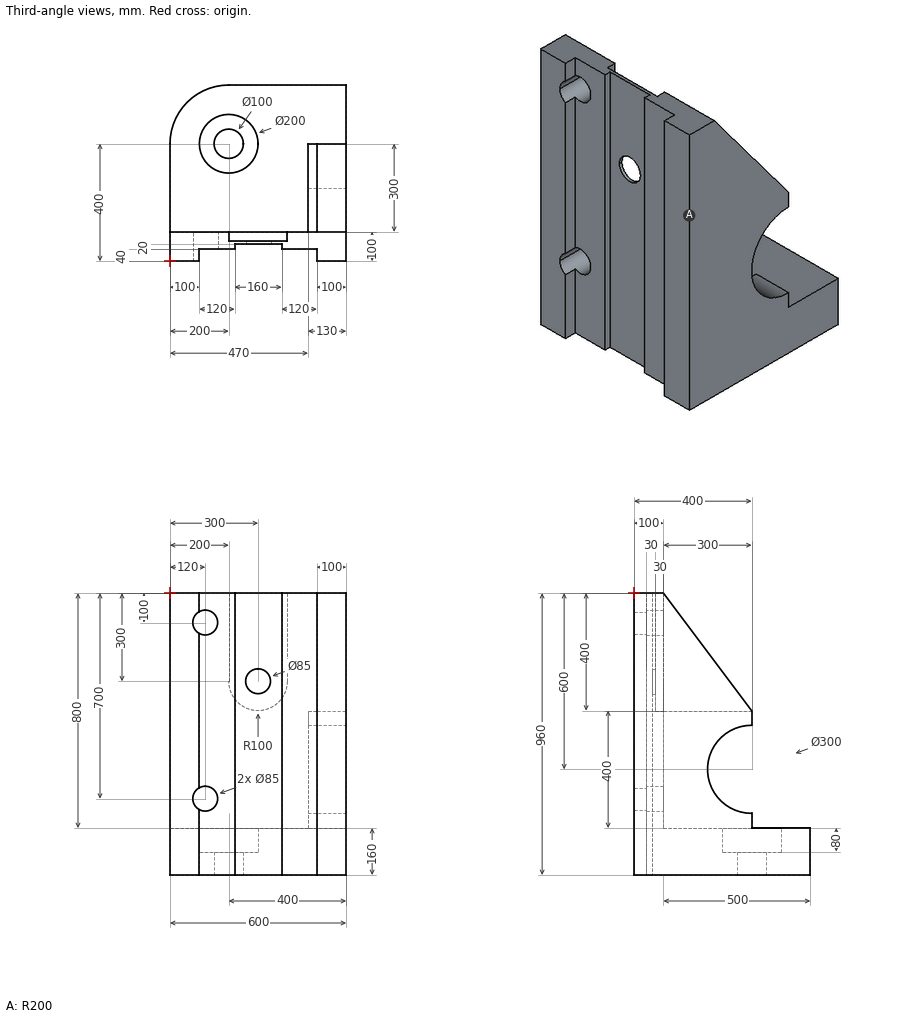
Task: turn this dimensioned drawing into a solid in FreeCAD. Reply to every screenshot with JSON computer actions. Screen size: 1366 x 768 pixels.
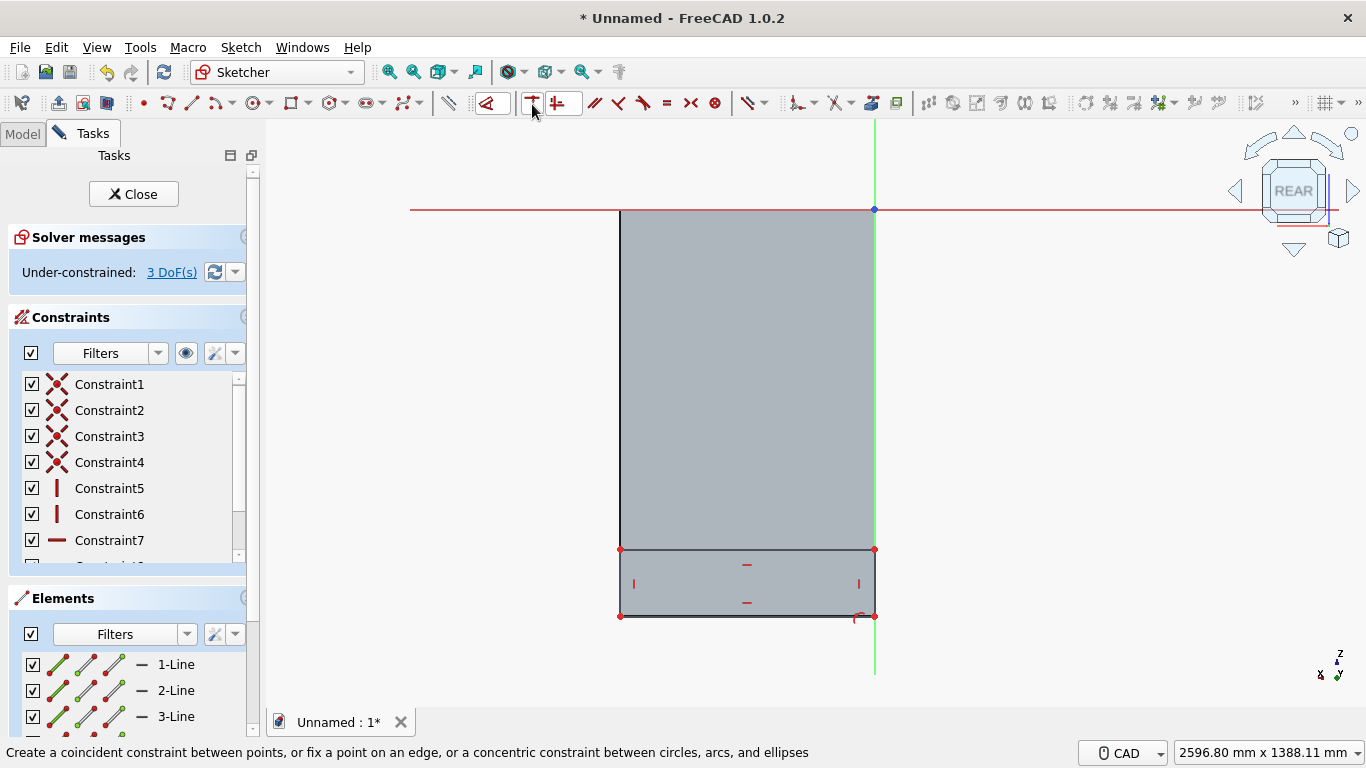
{"action": "left_click", "coordinate": [620, 570]}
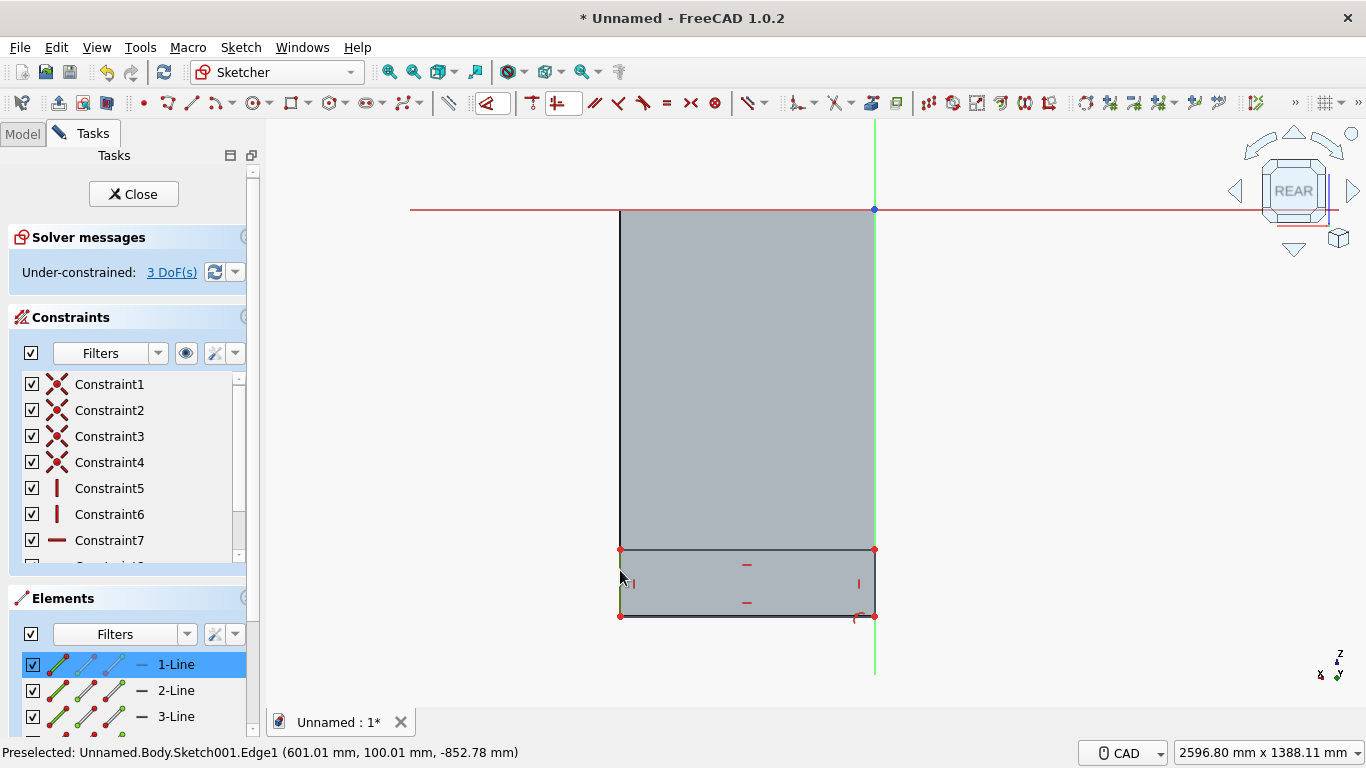
{"action": "left_click", "coordinate": [504, 104]}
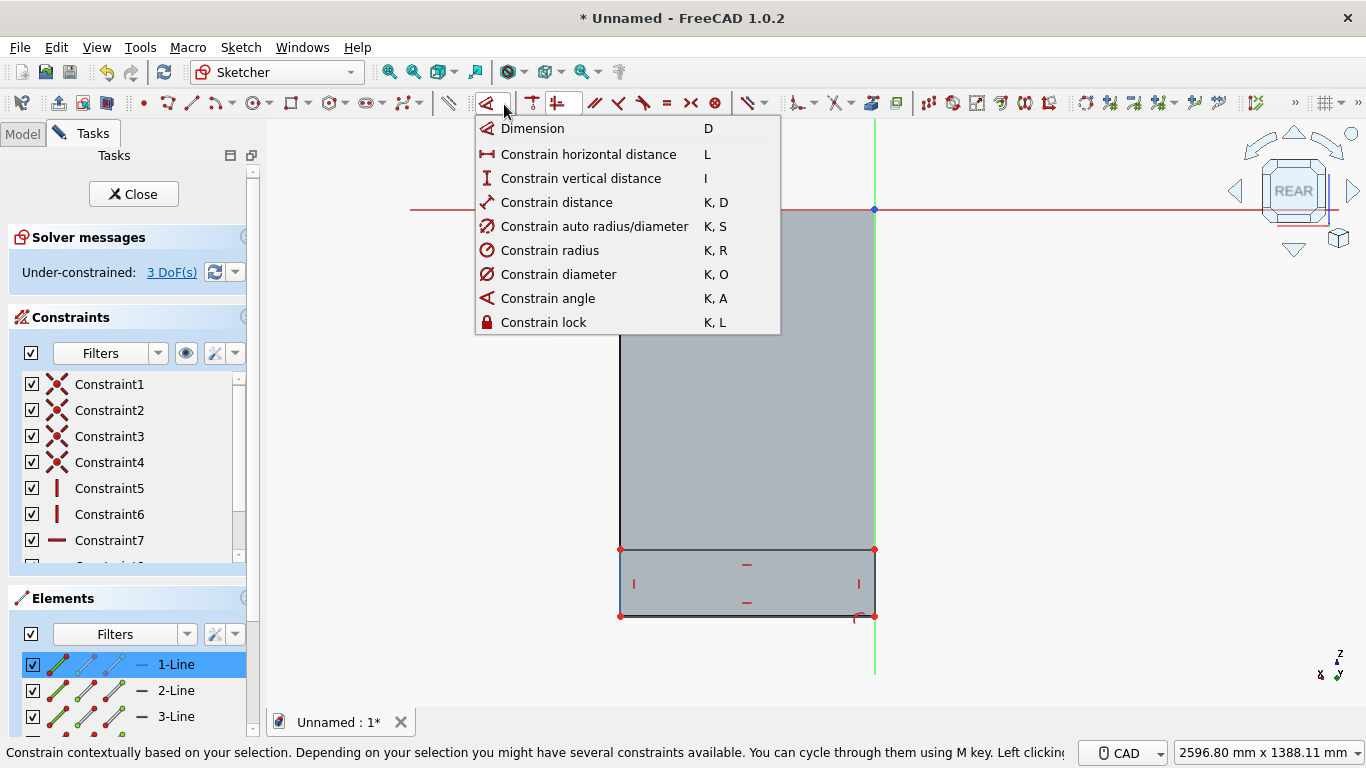
{"action": "left_click", "coordinate": [628, 178]}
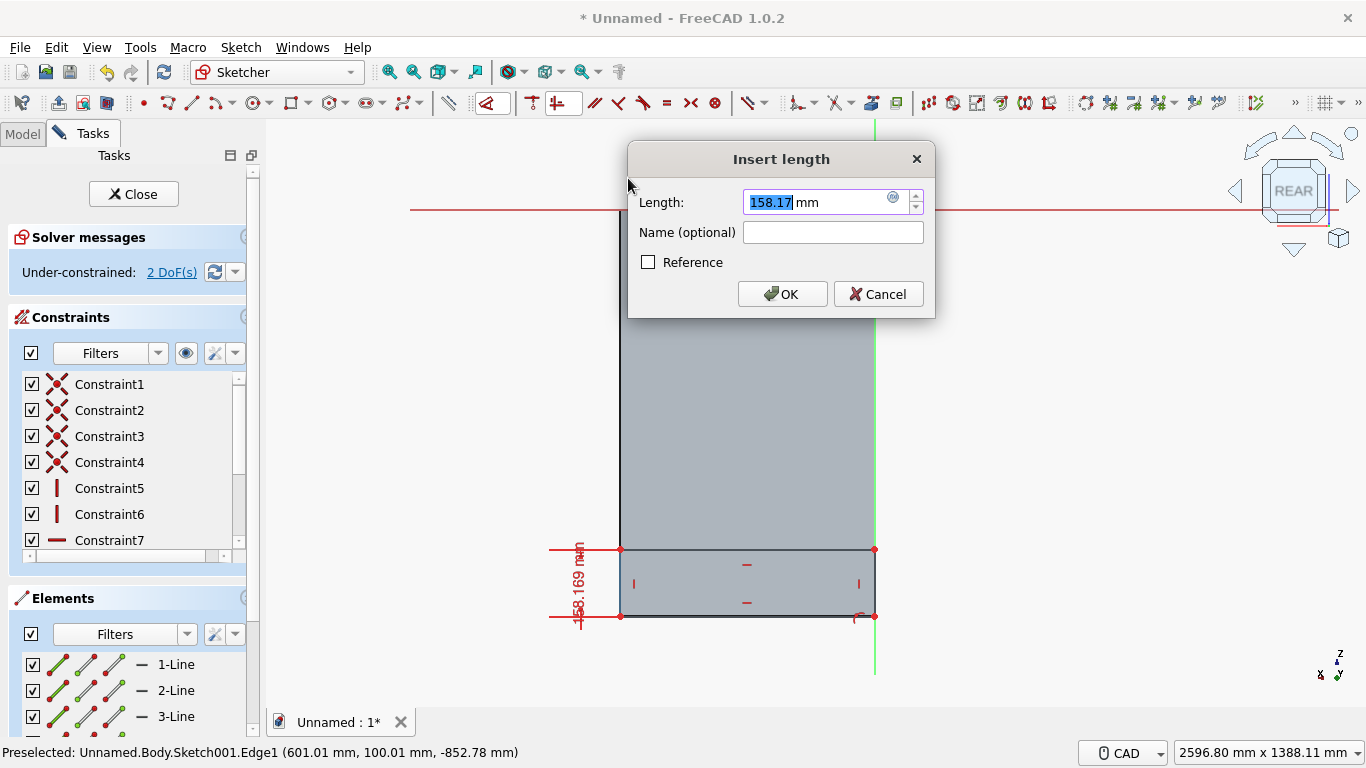
{"action": "type", "text": "160"}
{"action": "key", "text": "Return"}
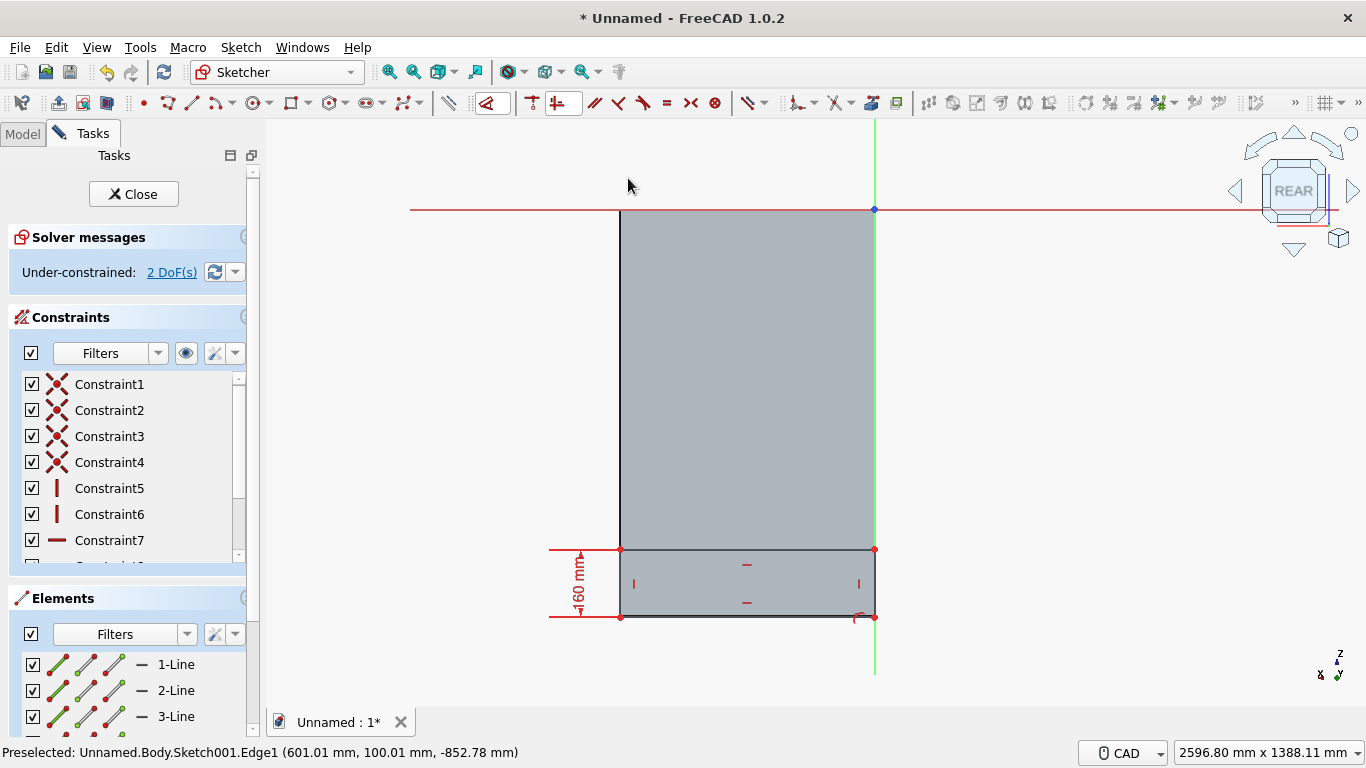
{"action": "left_click", "coordinate": [696, 617]}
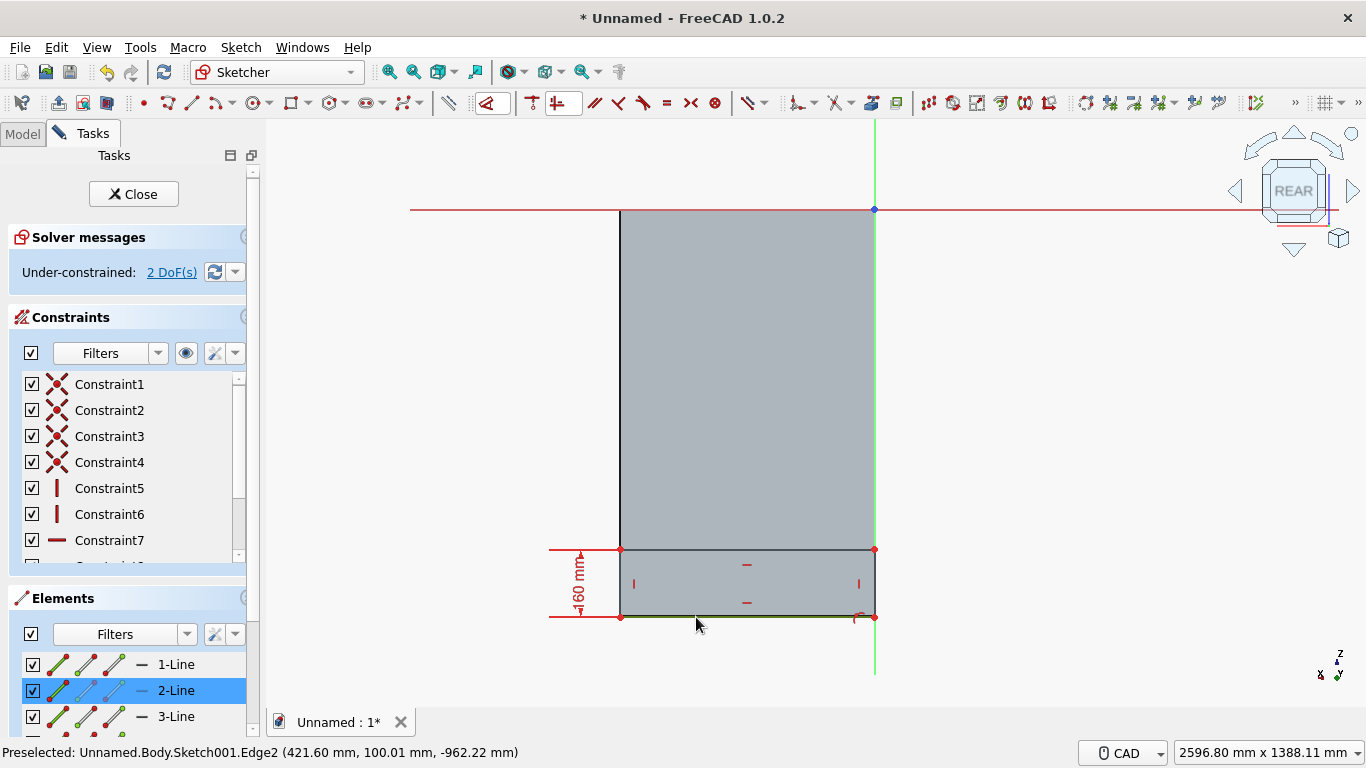
{"action": "left_click", "coordinate": [504, 104]}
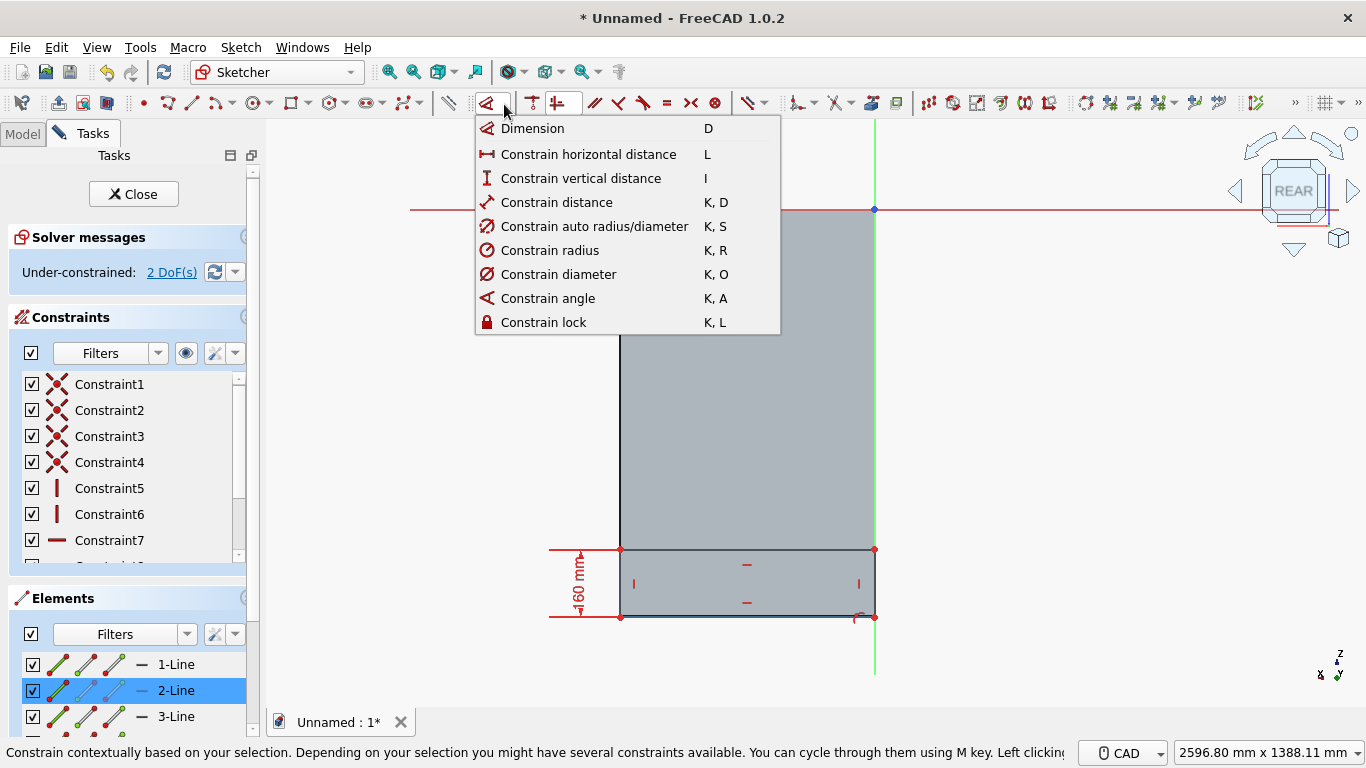
{"action": "left_click", "coordinate": [628, 154]}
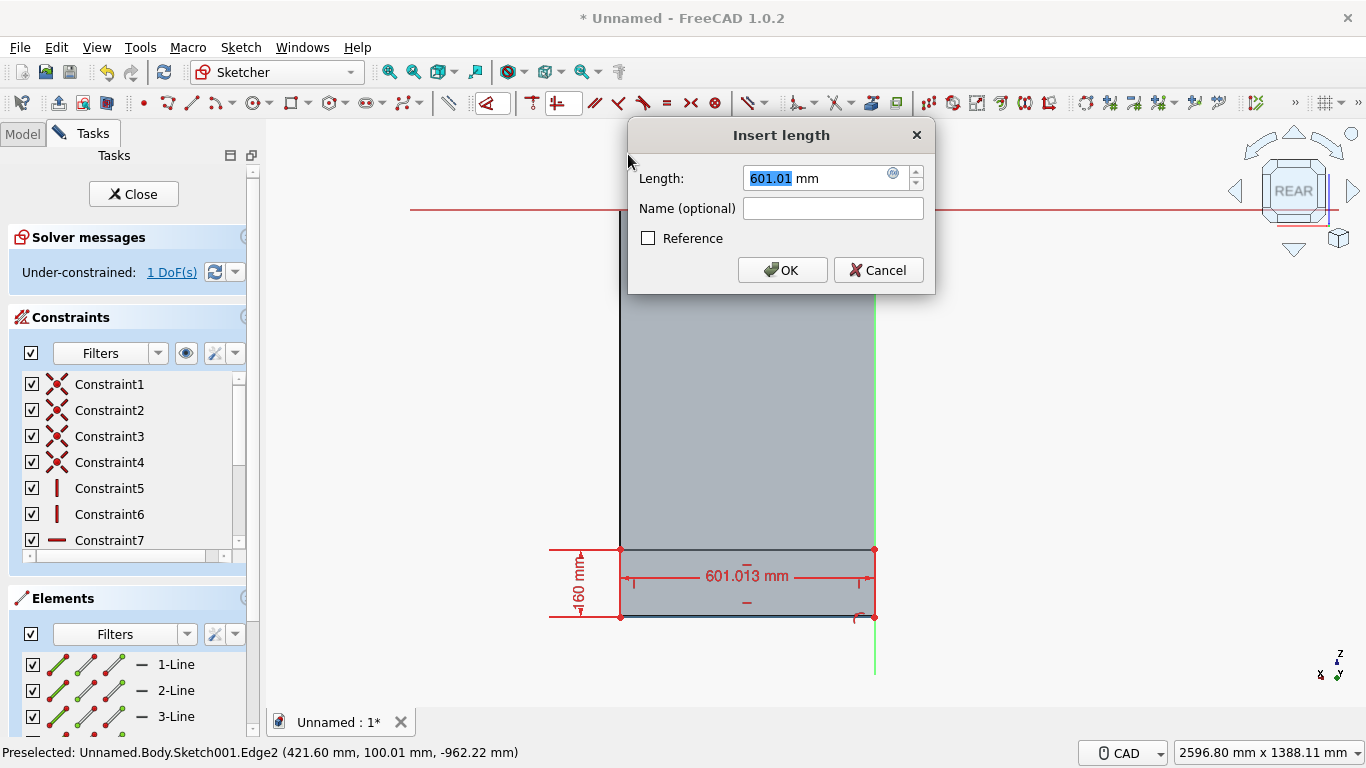
{"action": "type", "text": "600"}
{"action": "key", "text": "Return"}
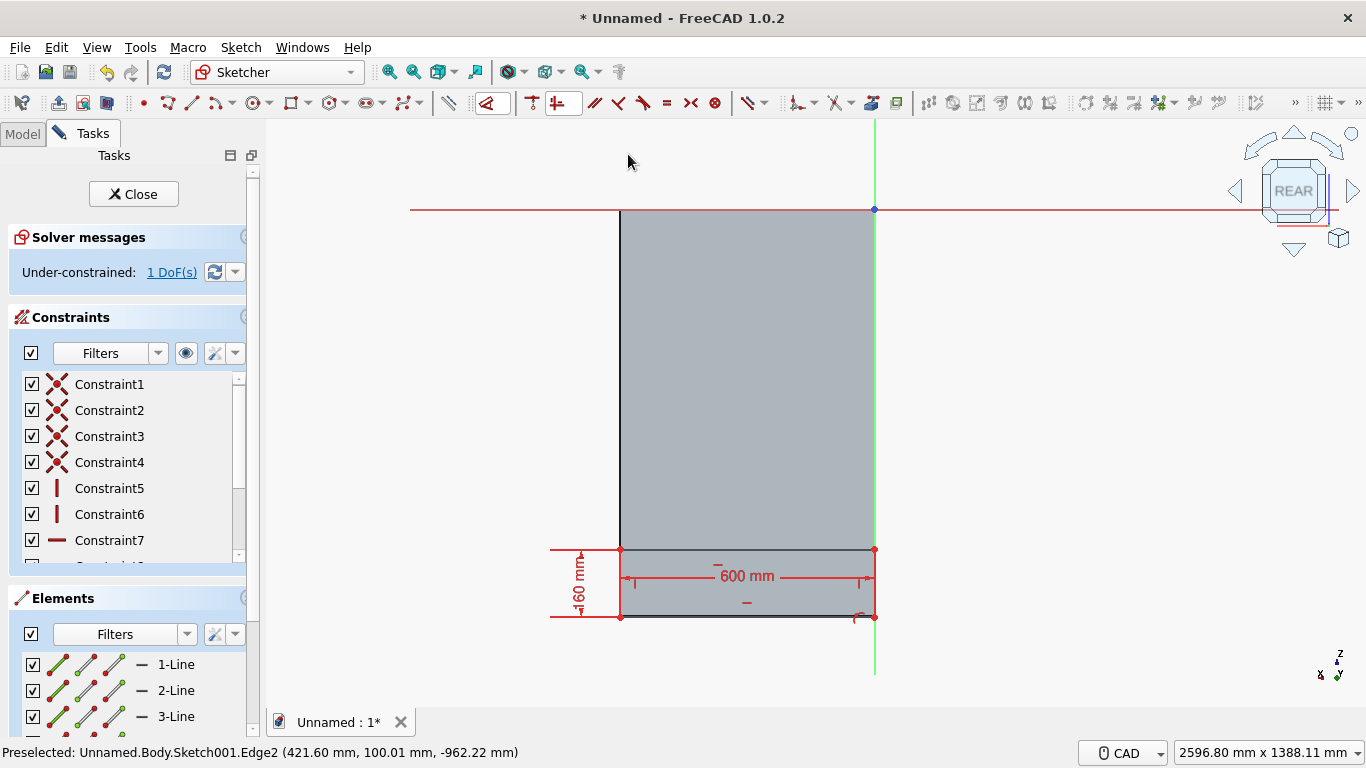
{"action": "left_click", "coordinate": [620, 550]}